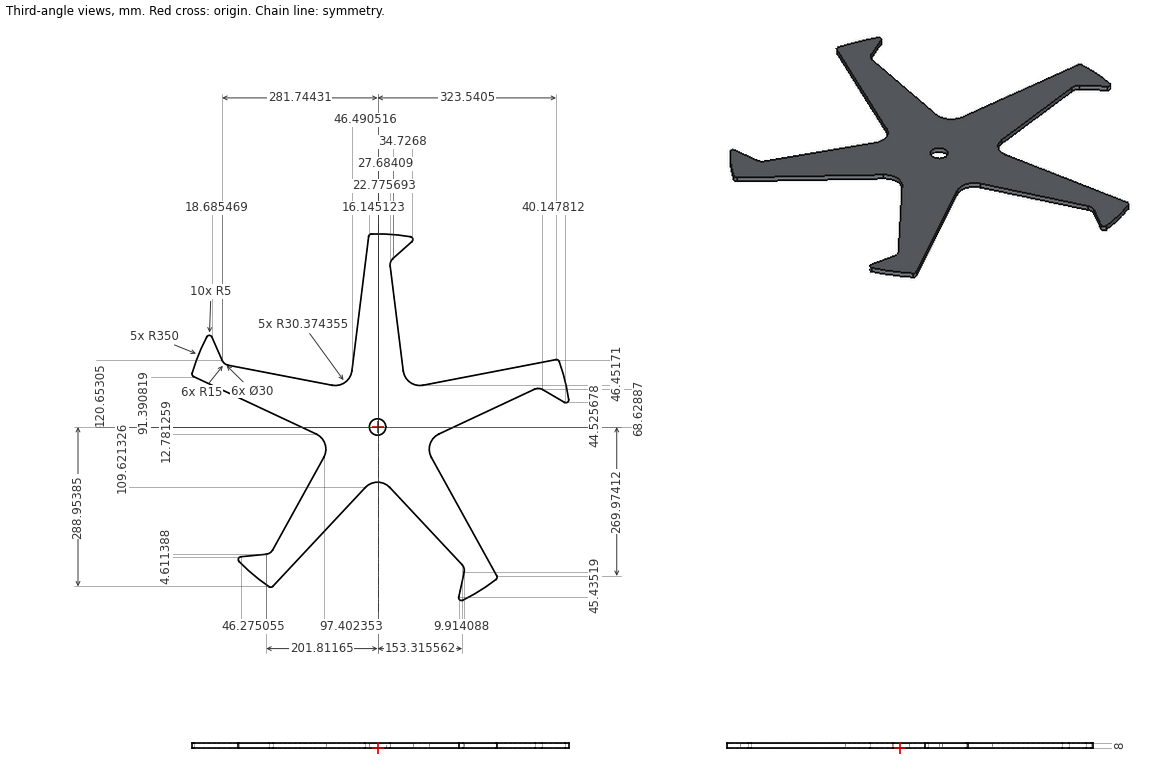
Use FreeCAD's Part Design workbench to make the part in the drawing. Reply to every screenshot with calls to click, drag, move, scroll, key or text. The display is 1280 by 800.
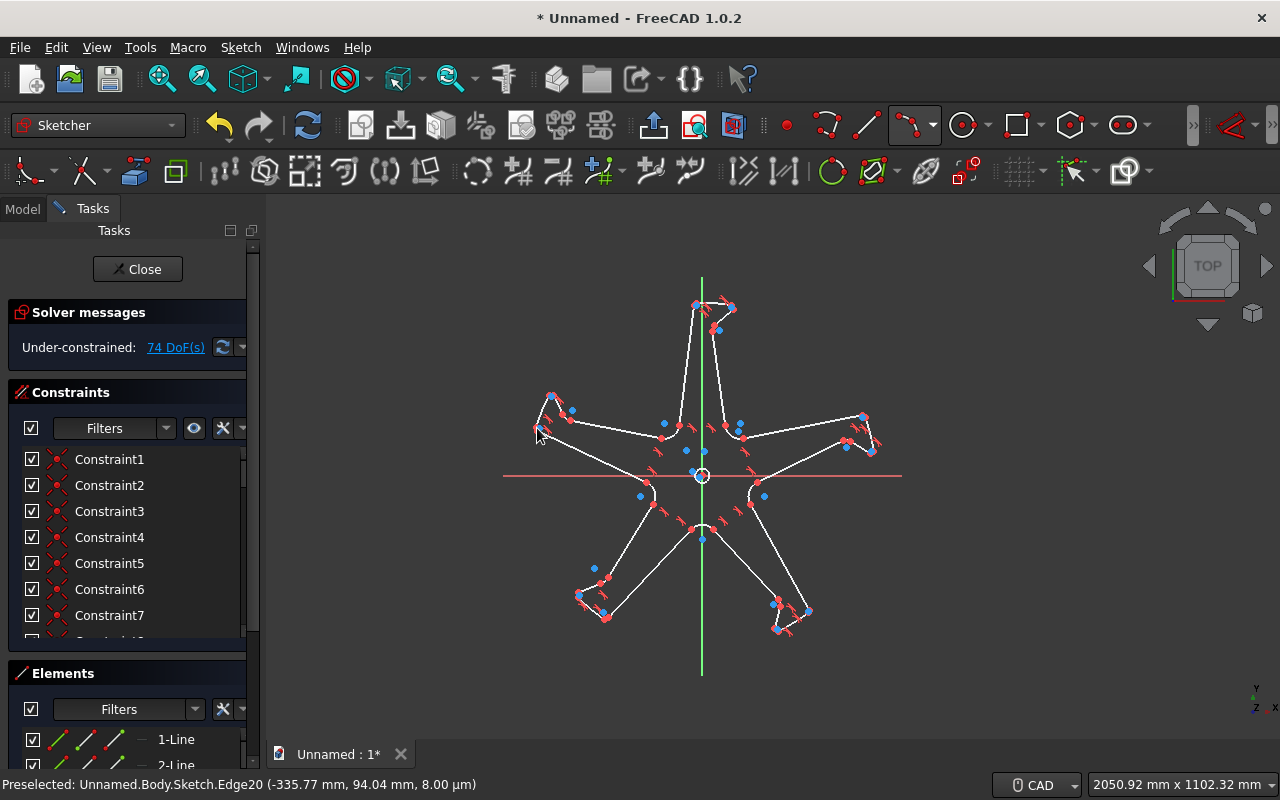
scroll(577, 594, up, 10)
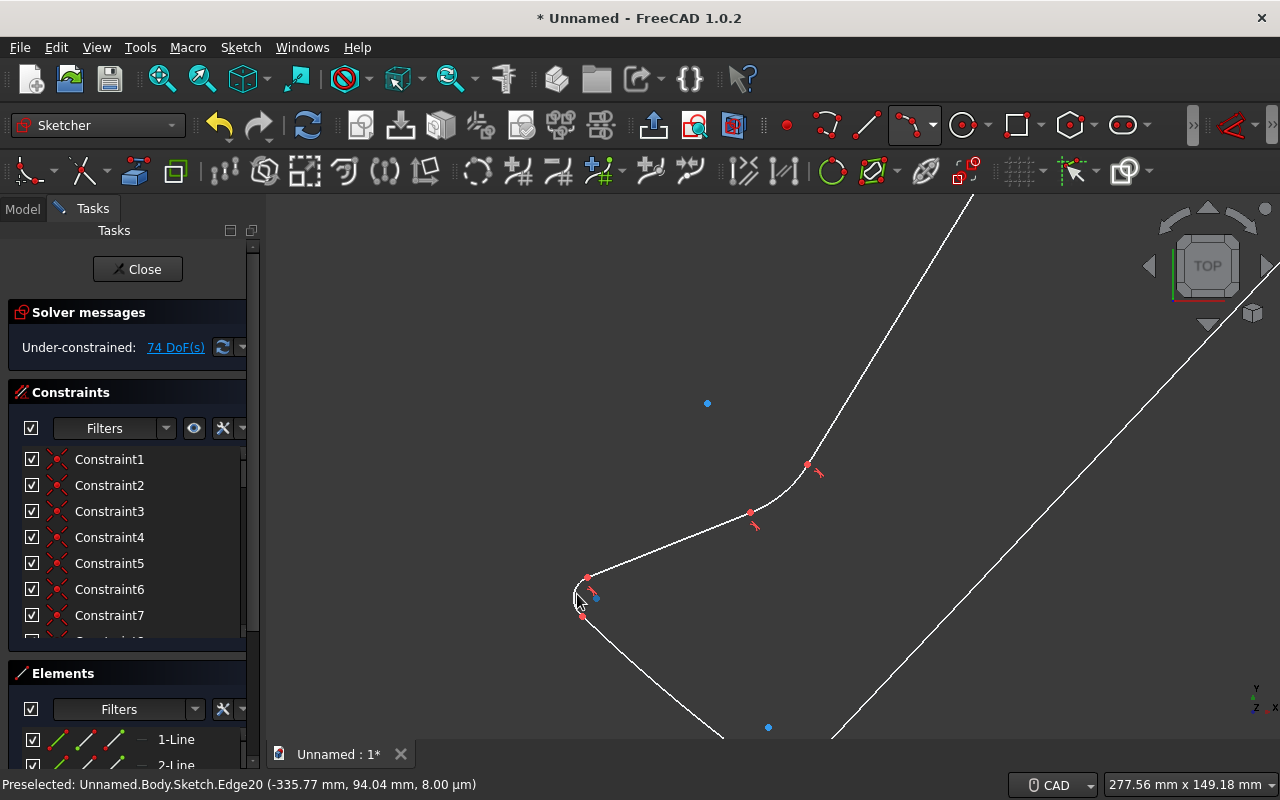
click(577, 586)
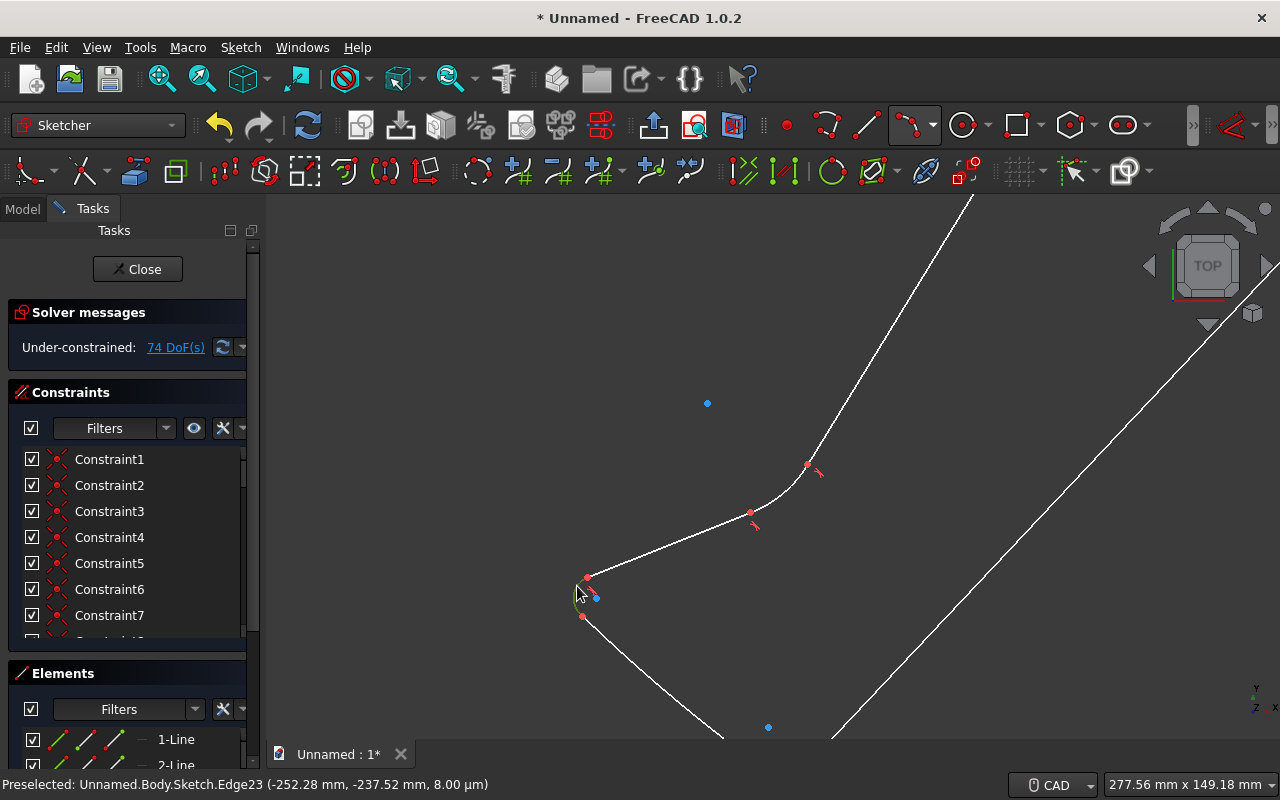
scroll(577, 594, down, 10)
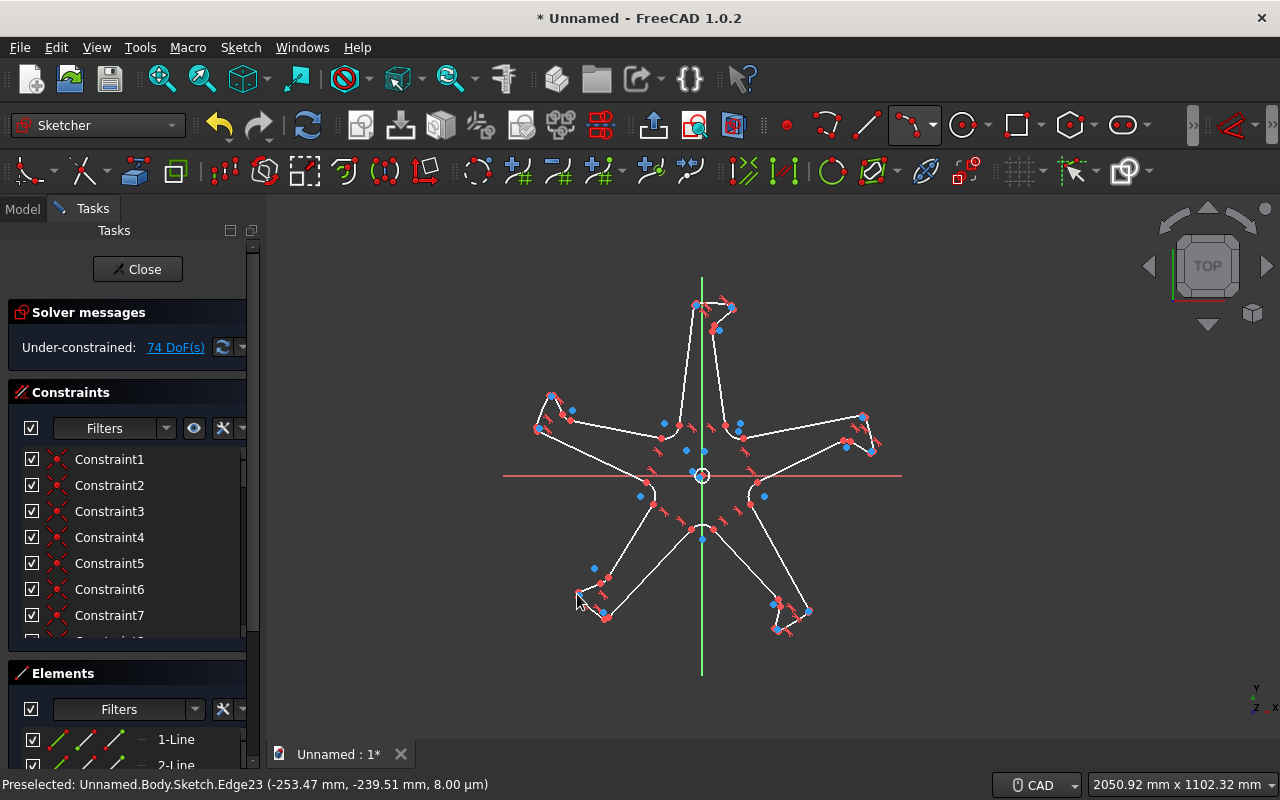
scroll(586, 605, up, 2)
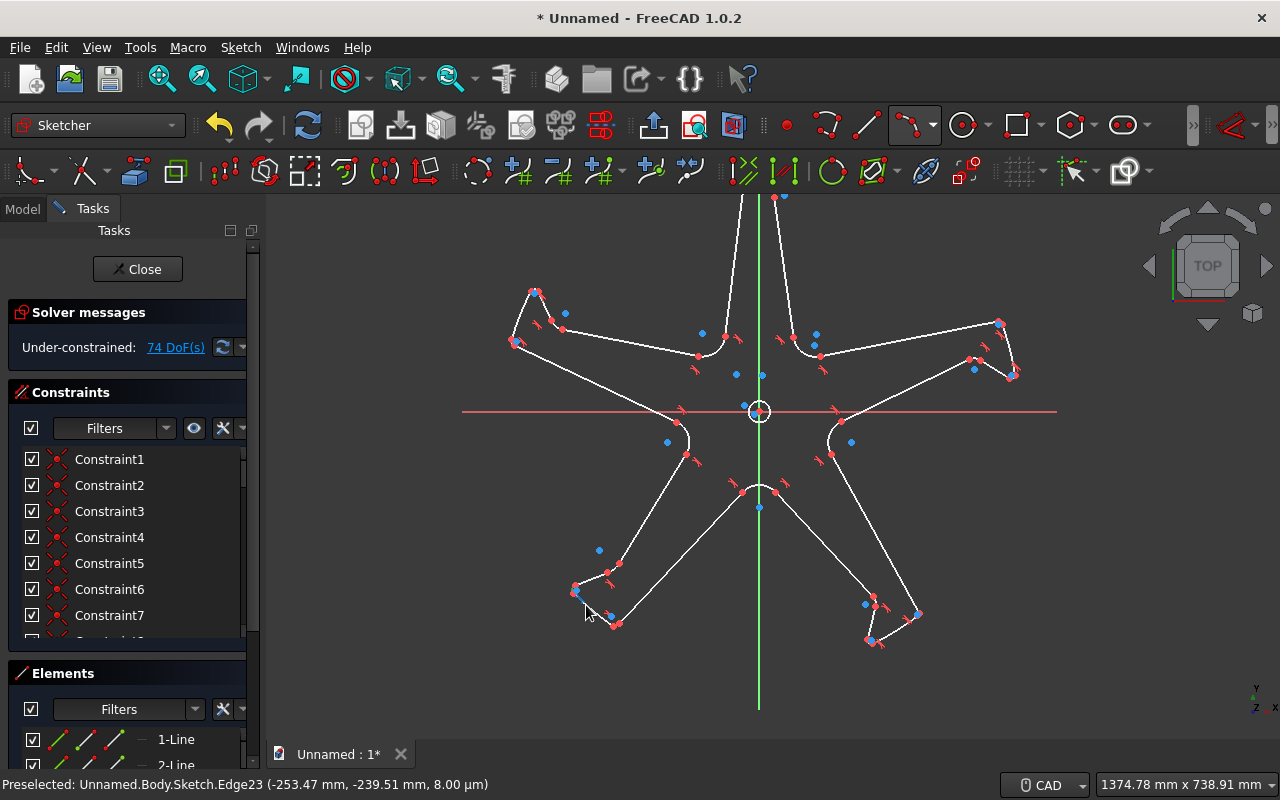
click(585, 604)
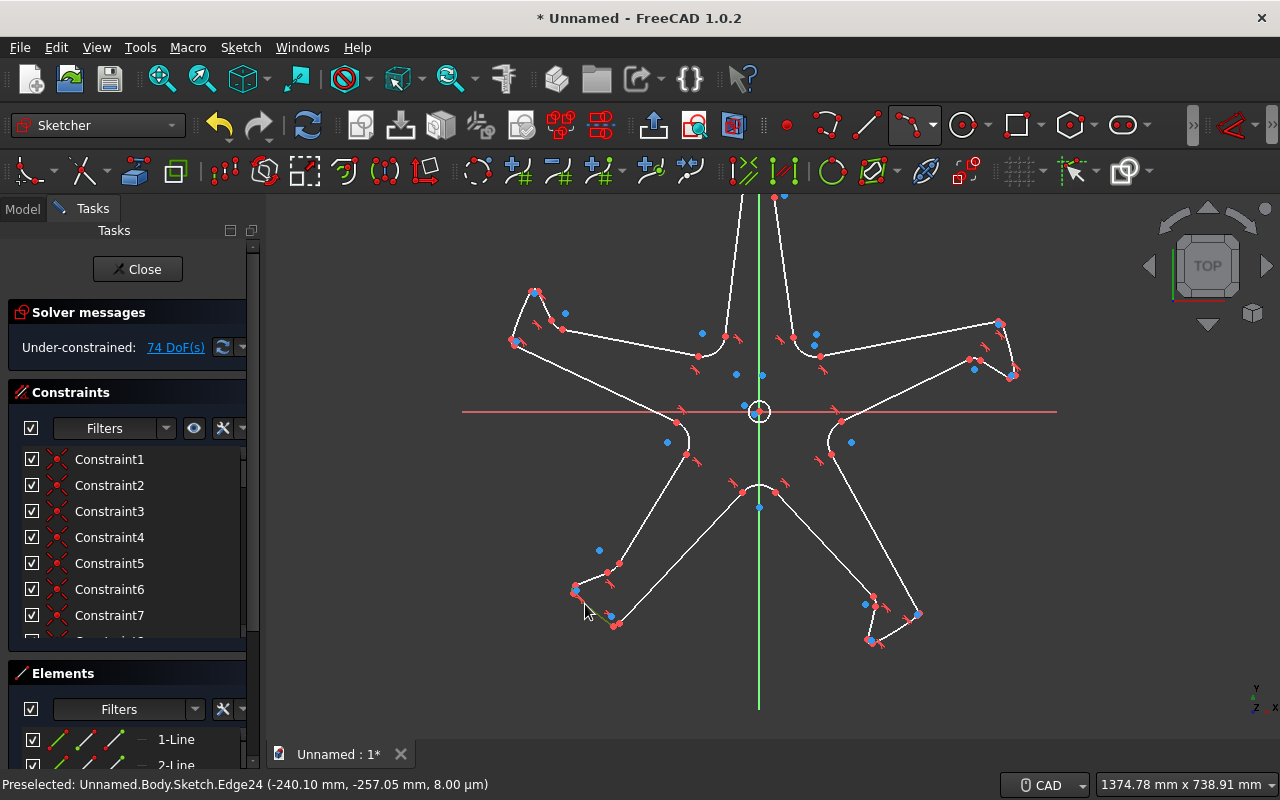
key(t)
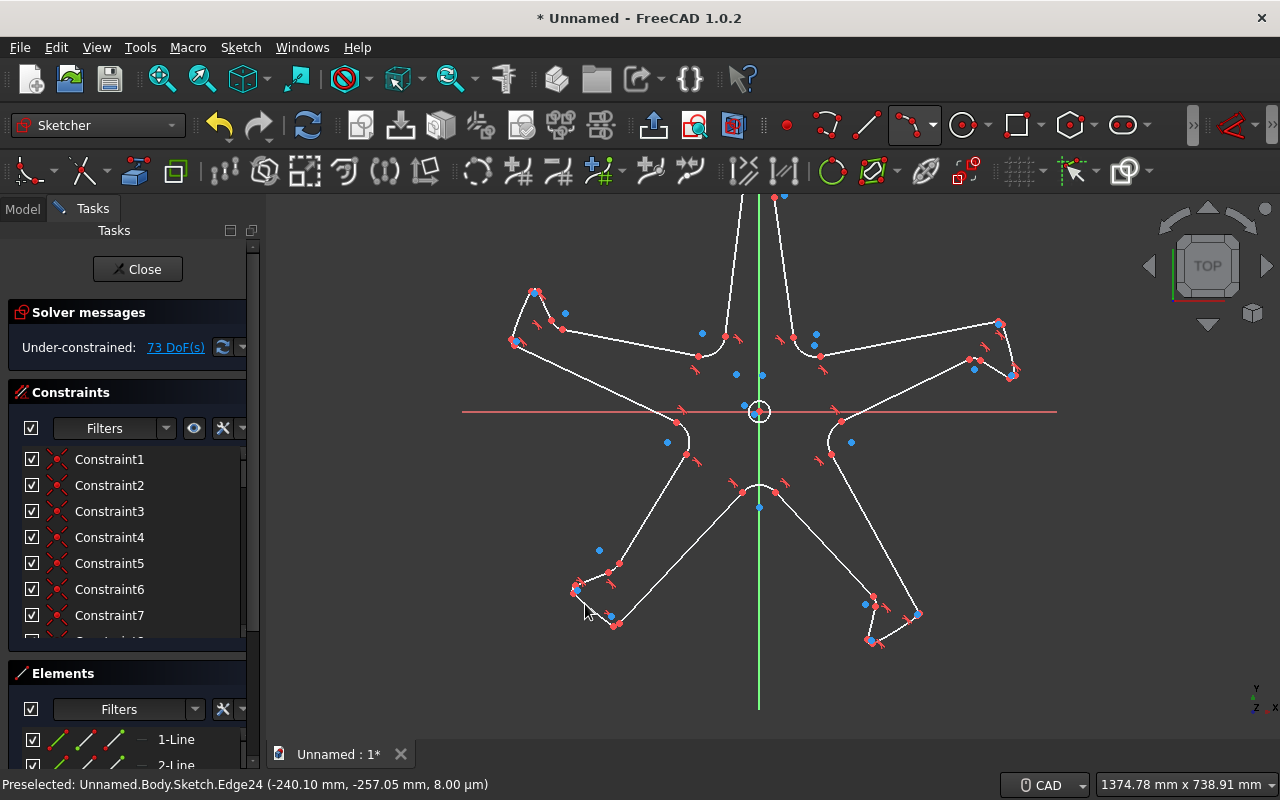
click(585, 604)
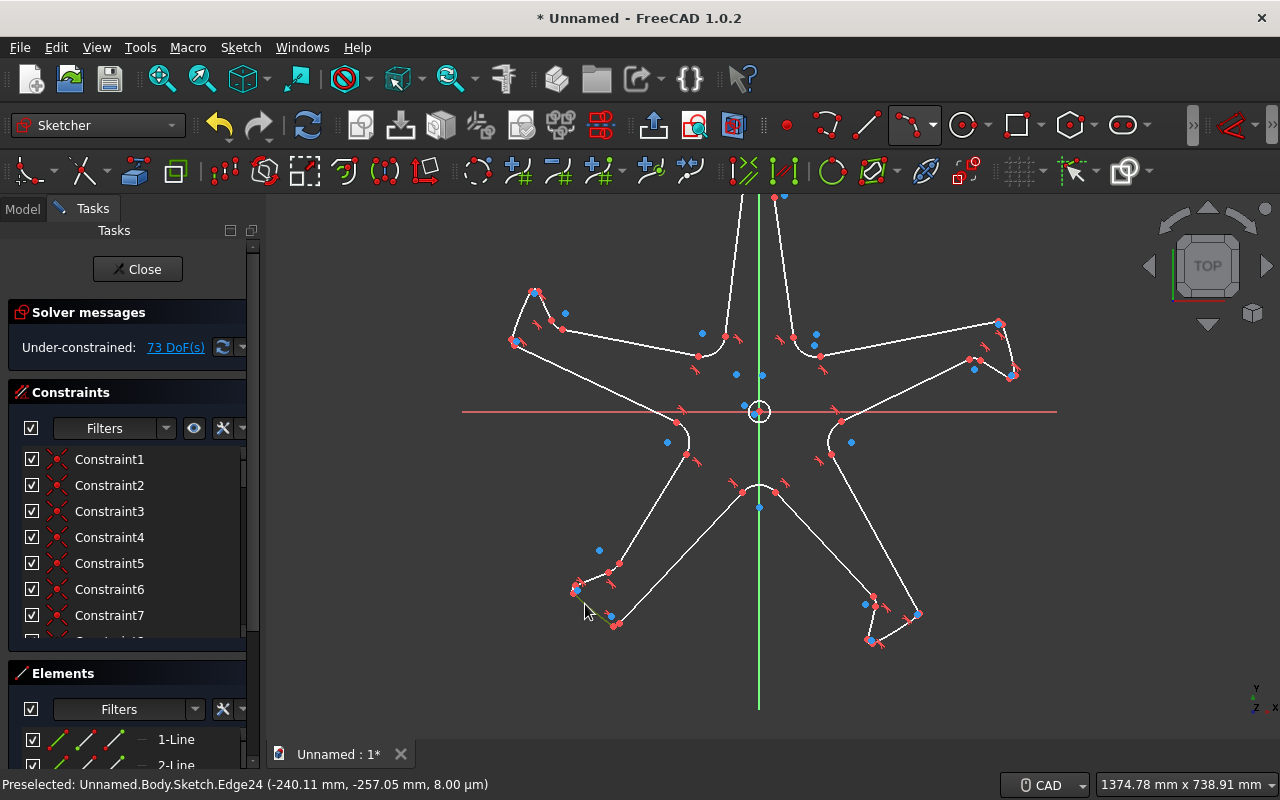
scroll(617, 626, up, 8)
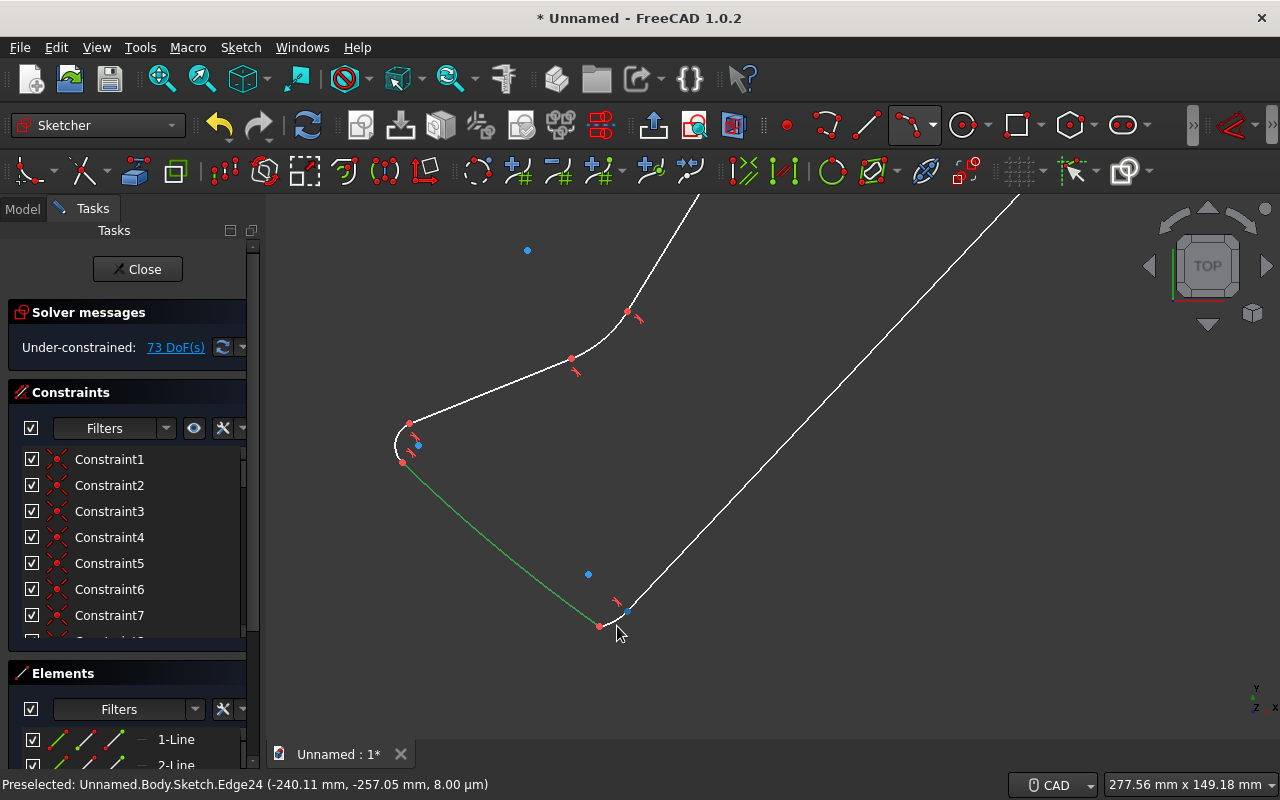
click(615, 621)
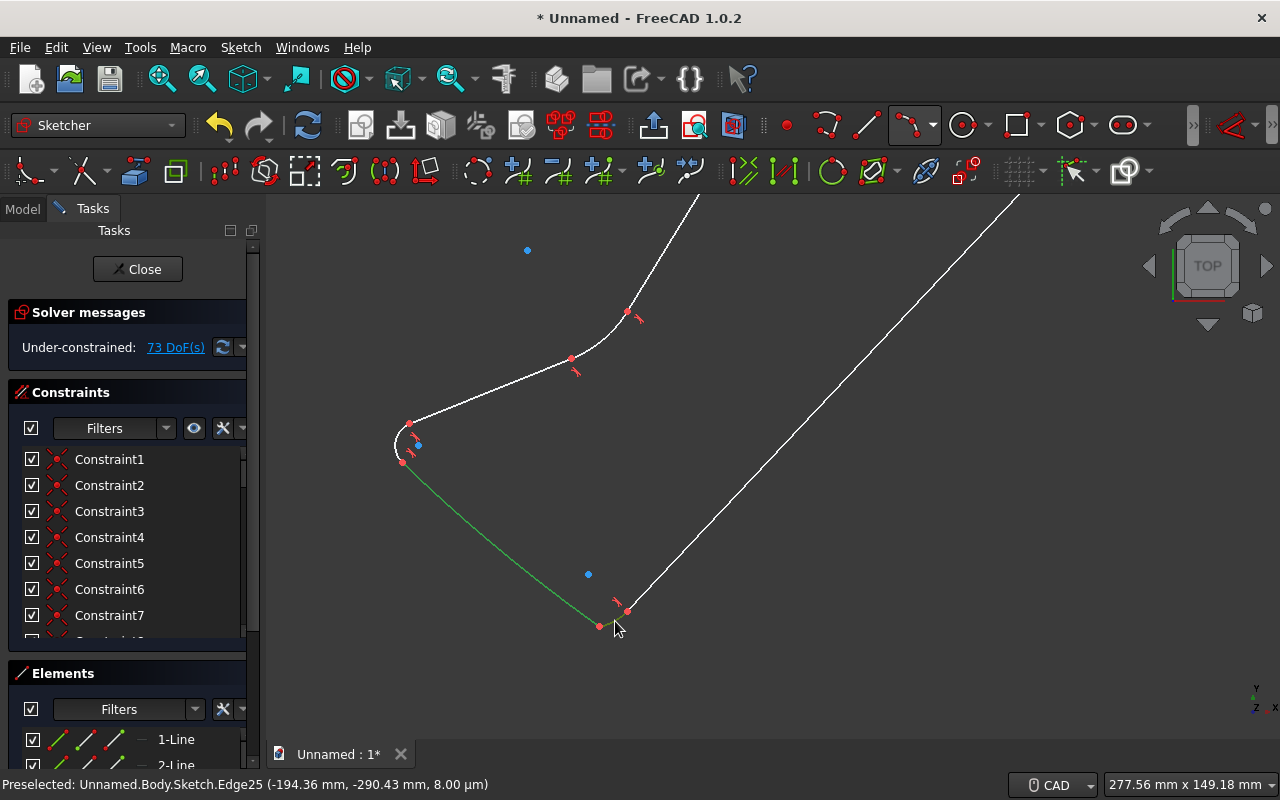
key(t)